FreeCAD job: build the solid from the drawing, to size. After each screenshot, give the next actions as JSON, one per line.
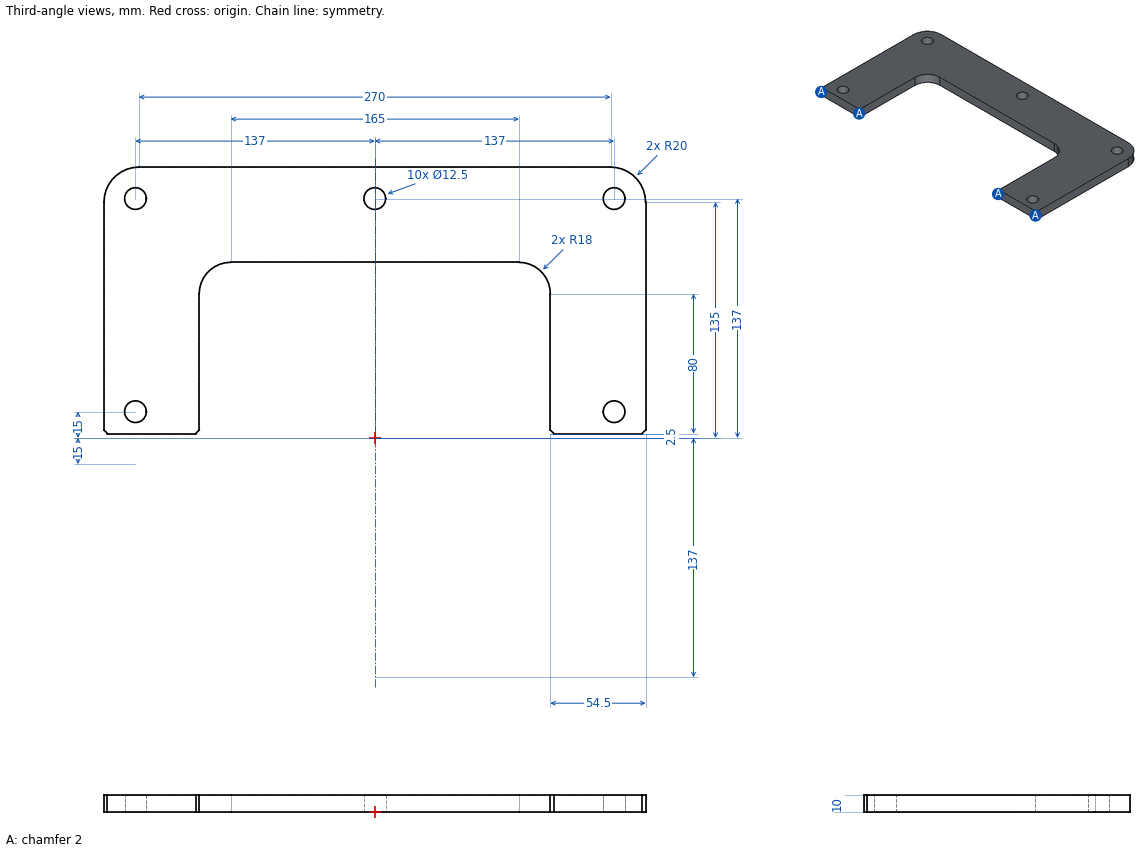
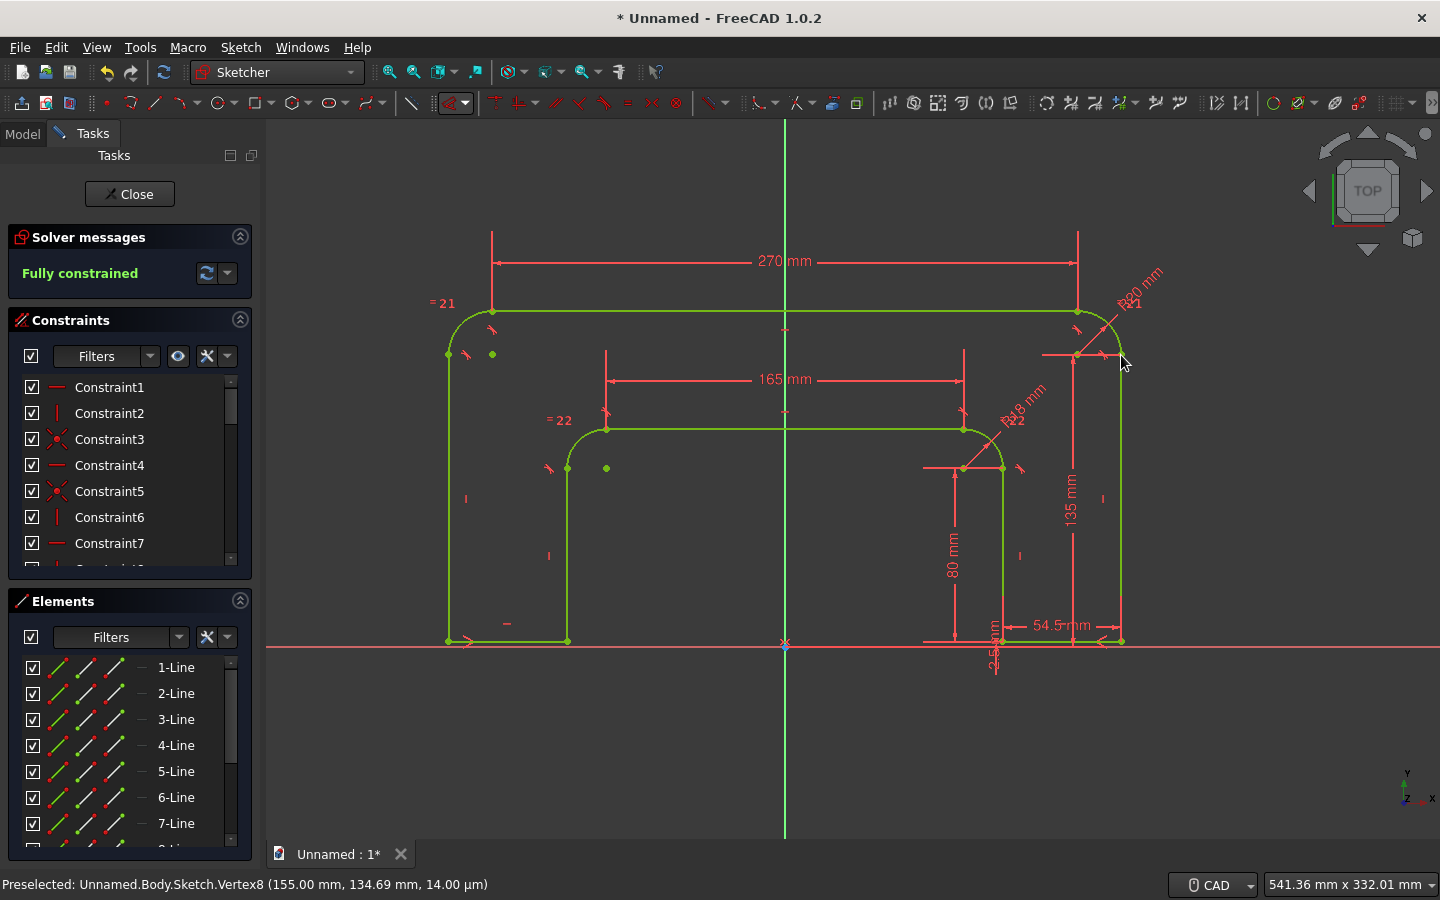
{"action": "left_click", "coordinate": [130, 194]}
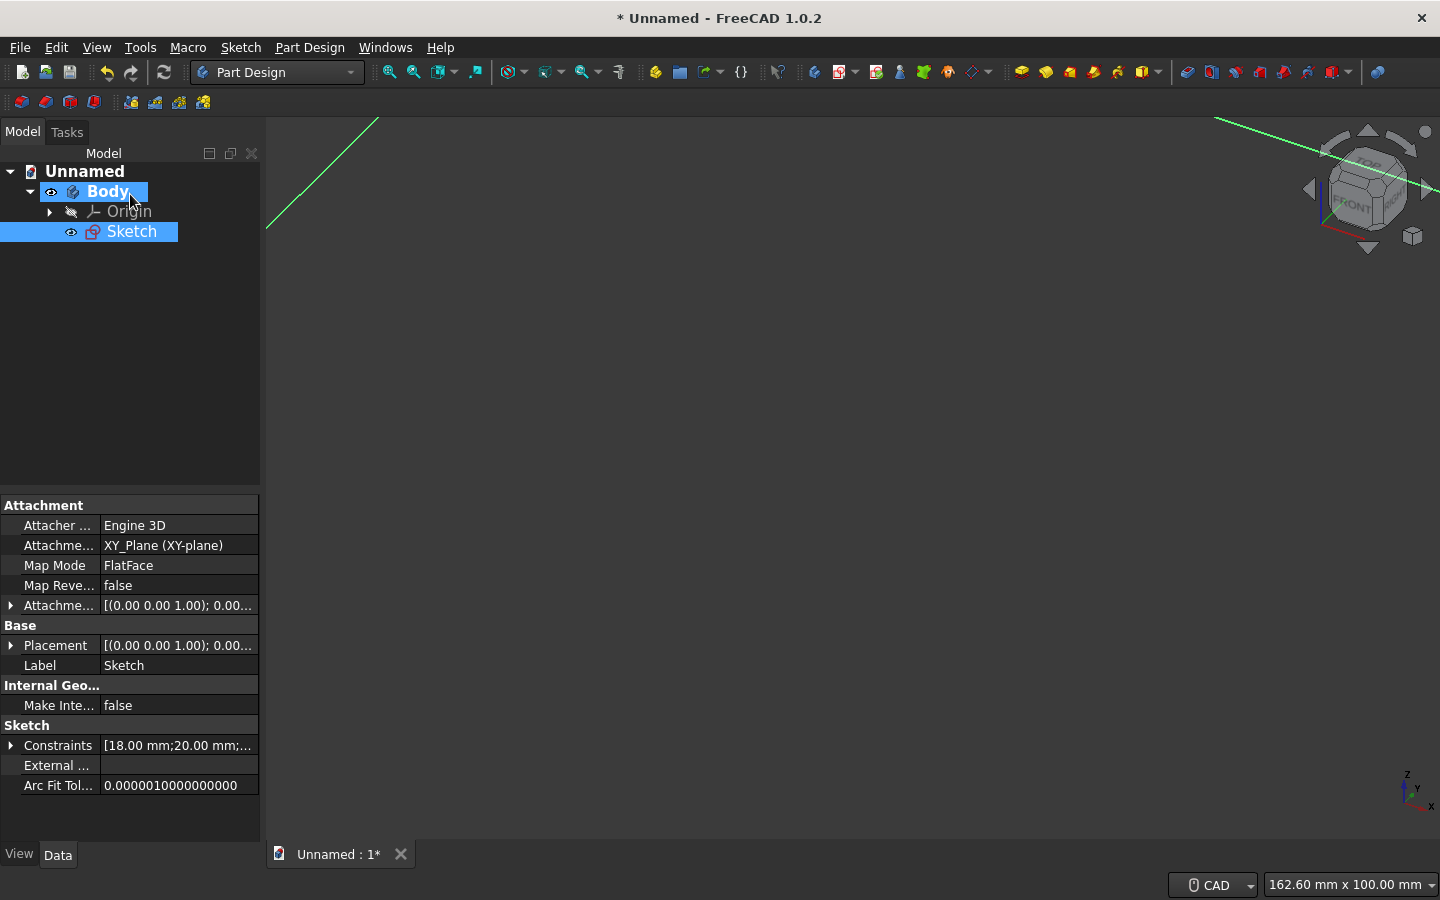
{"action": "left_click", "coordinate": [1022, 72]}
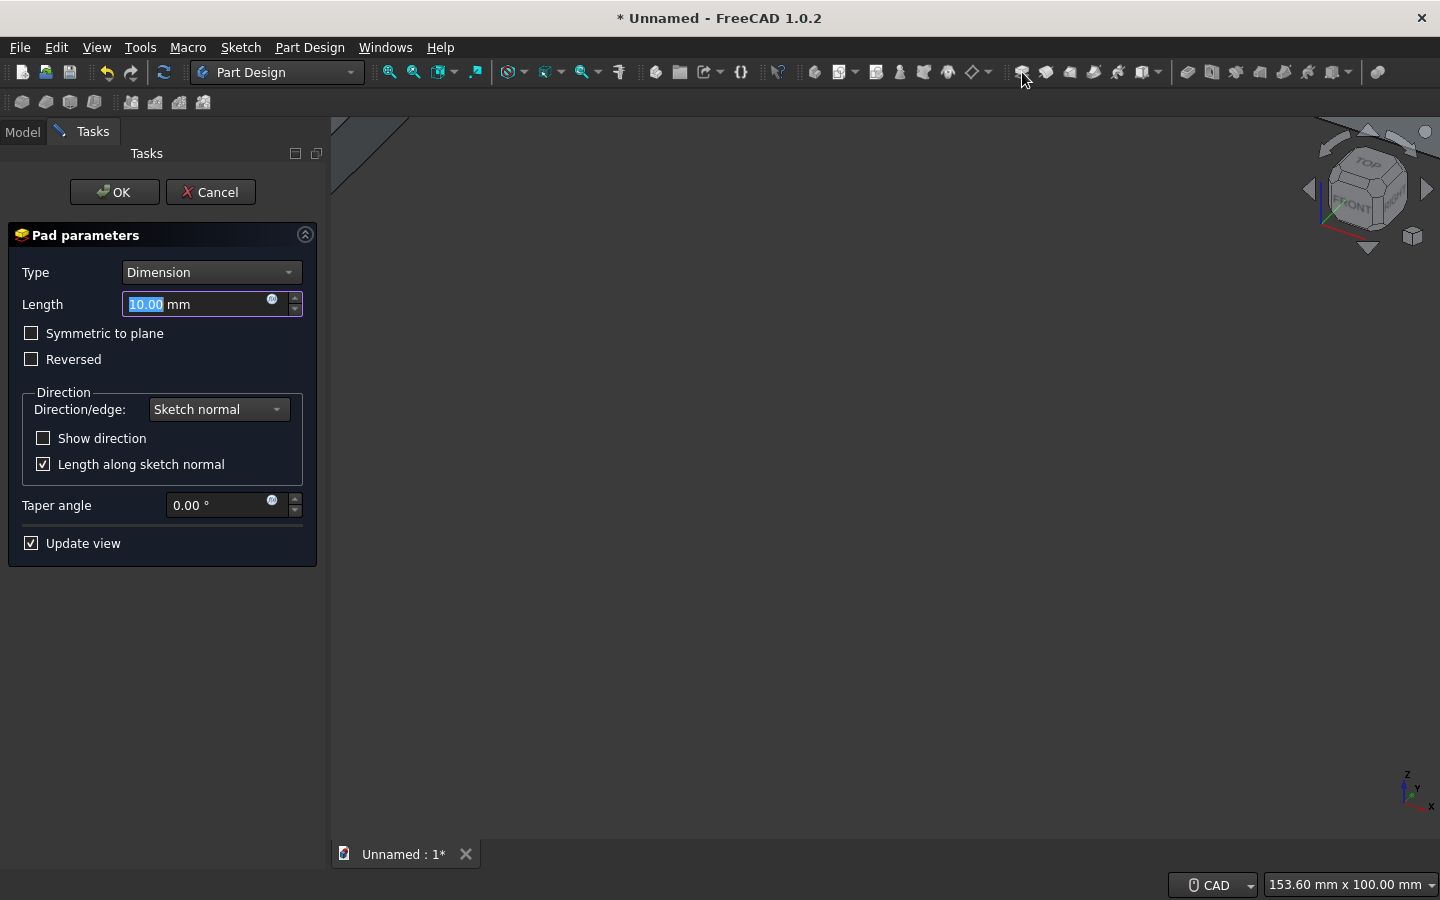
{"action": "type", "text": "10"}
{"action": "key", "text": "Tab"}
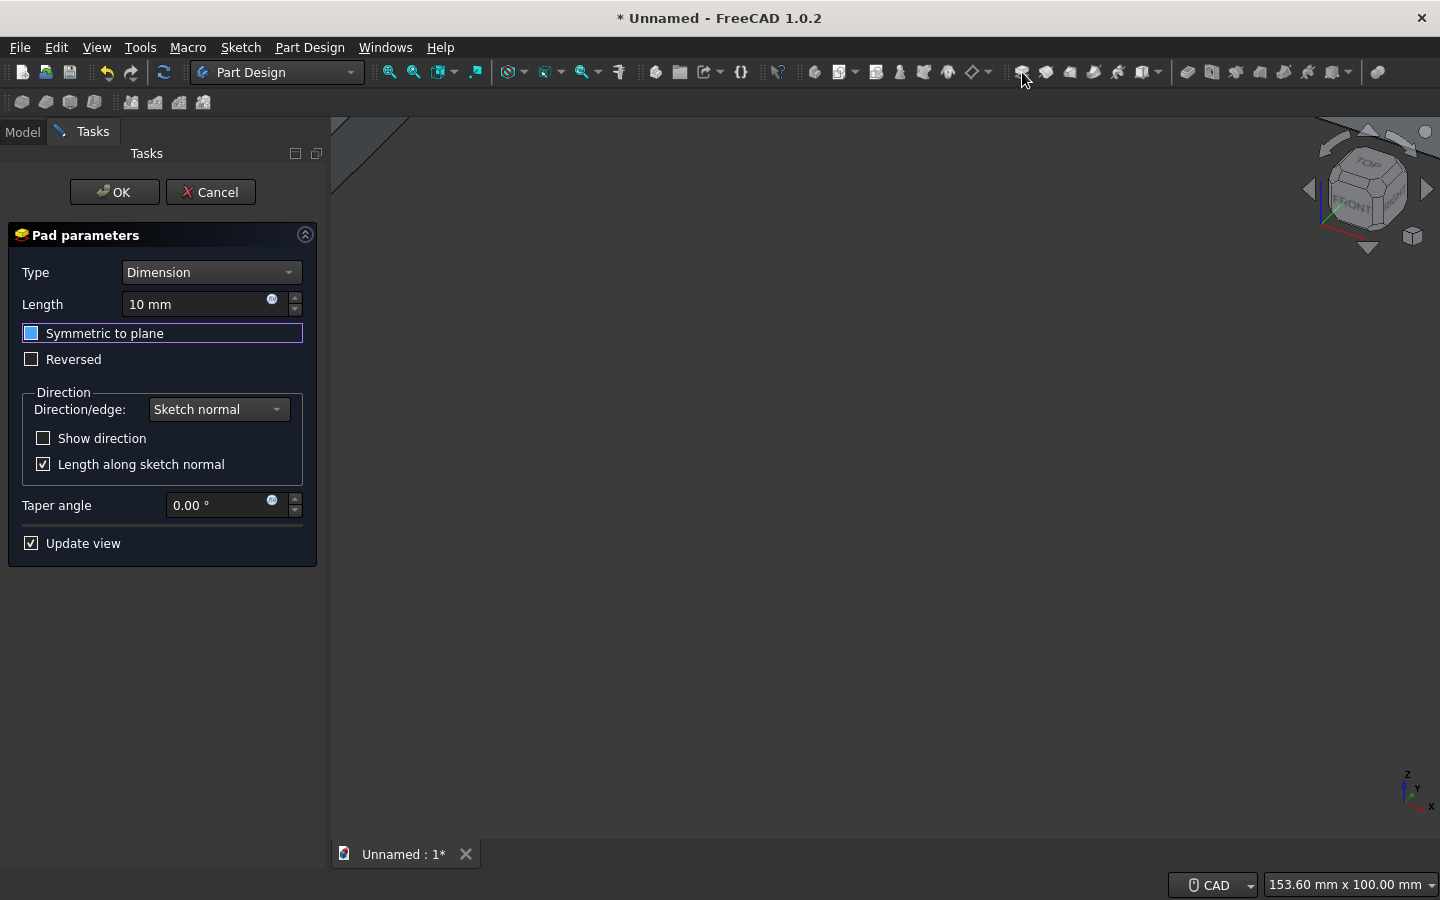
{"action": "left_click", "coordinate": [115, 192]}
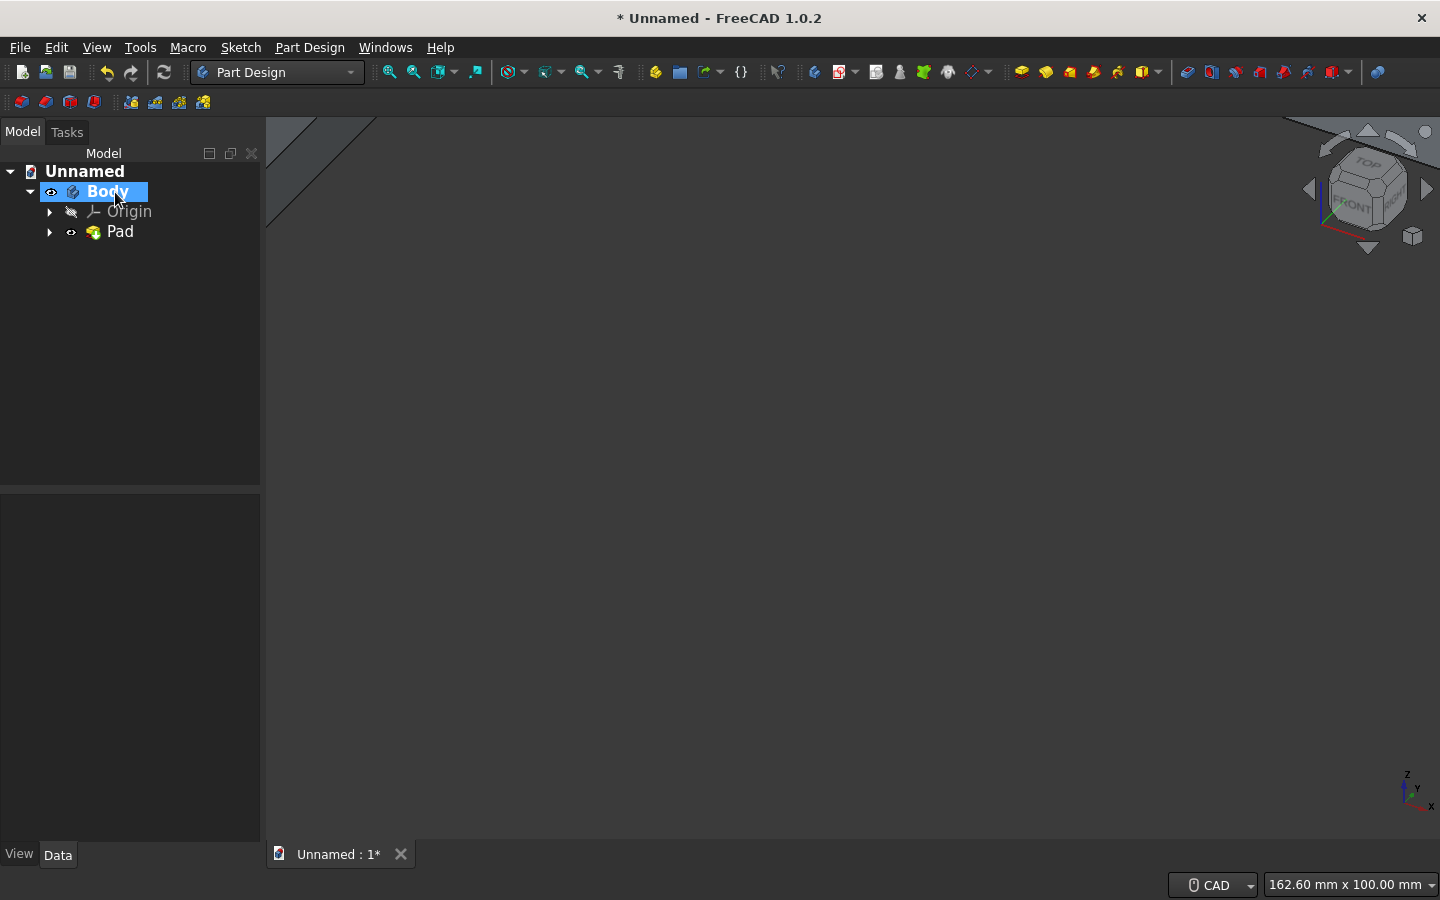
{"action": "left_click", "coordinate": [390, 72]}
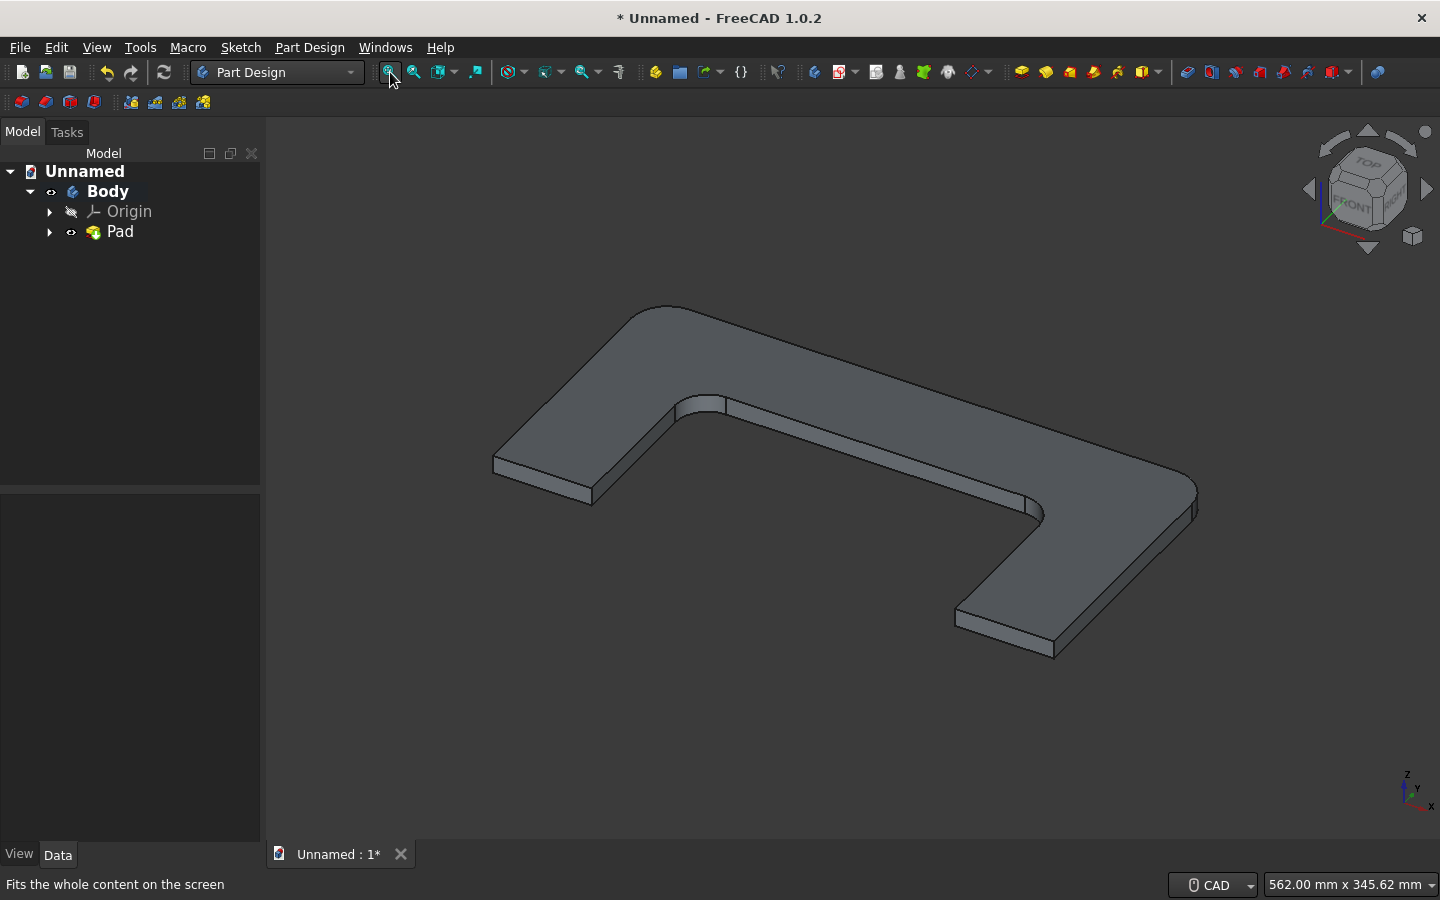
{"action": "left_click", "coordinate": [1059, 476]}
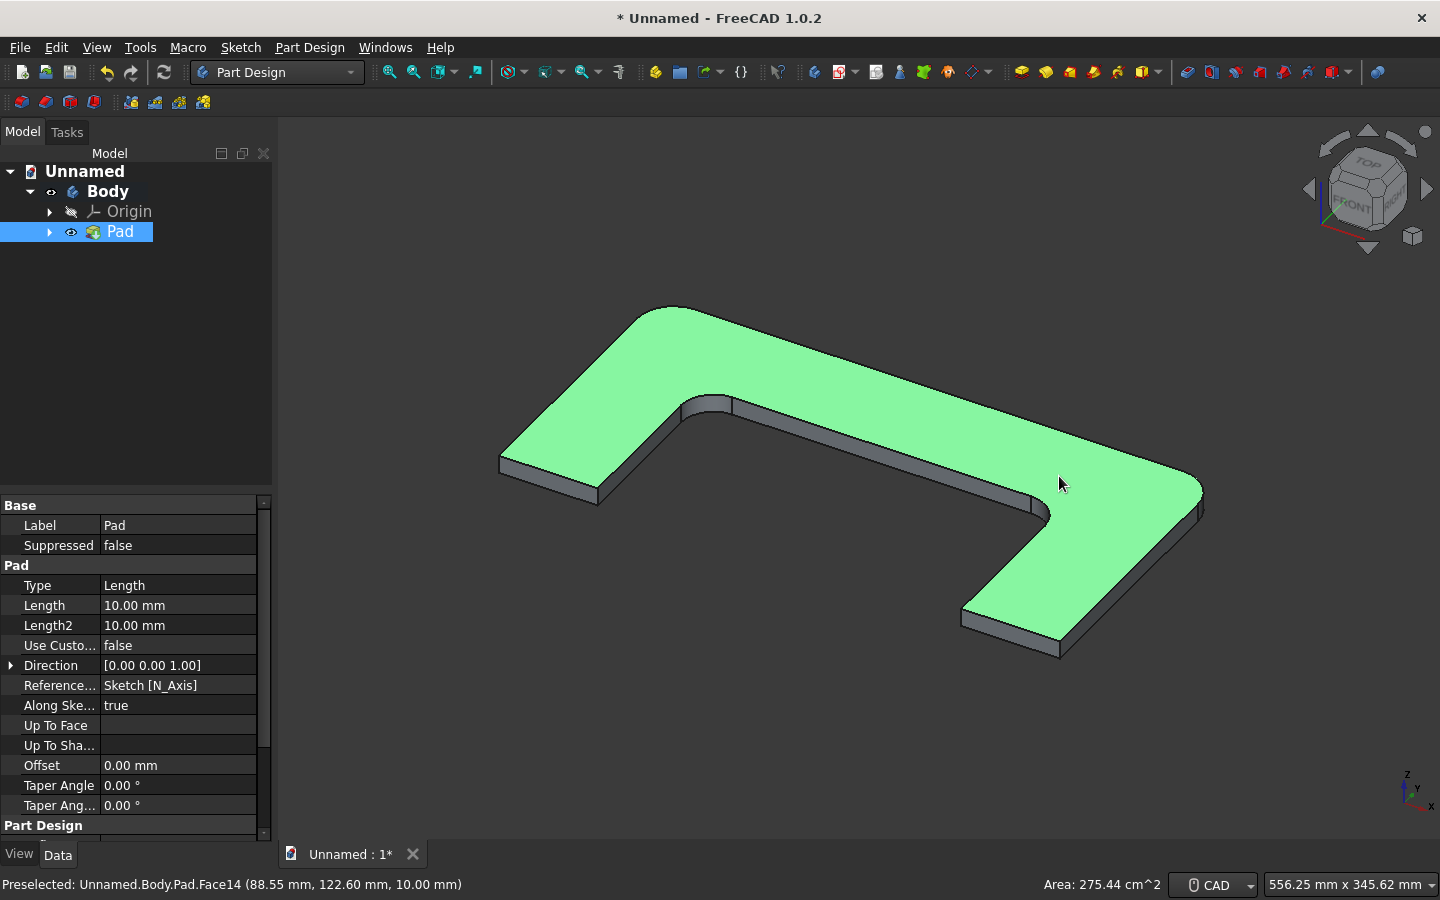
{"action": "left_click", "coordinate": [840, 72]}